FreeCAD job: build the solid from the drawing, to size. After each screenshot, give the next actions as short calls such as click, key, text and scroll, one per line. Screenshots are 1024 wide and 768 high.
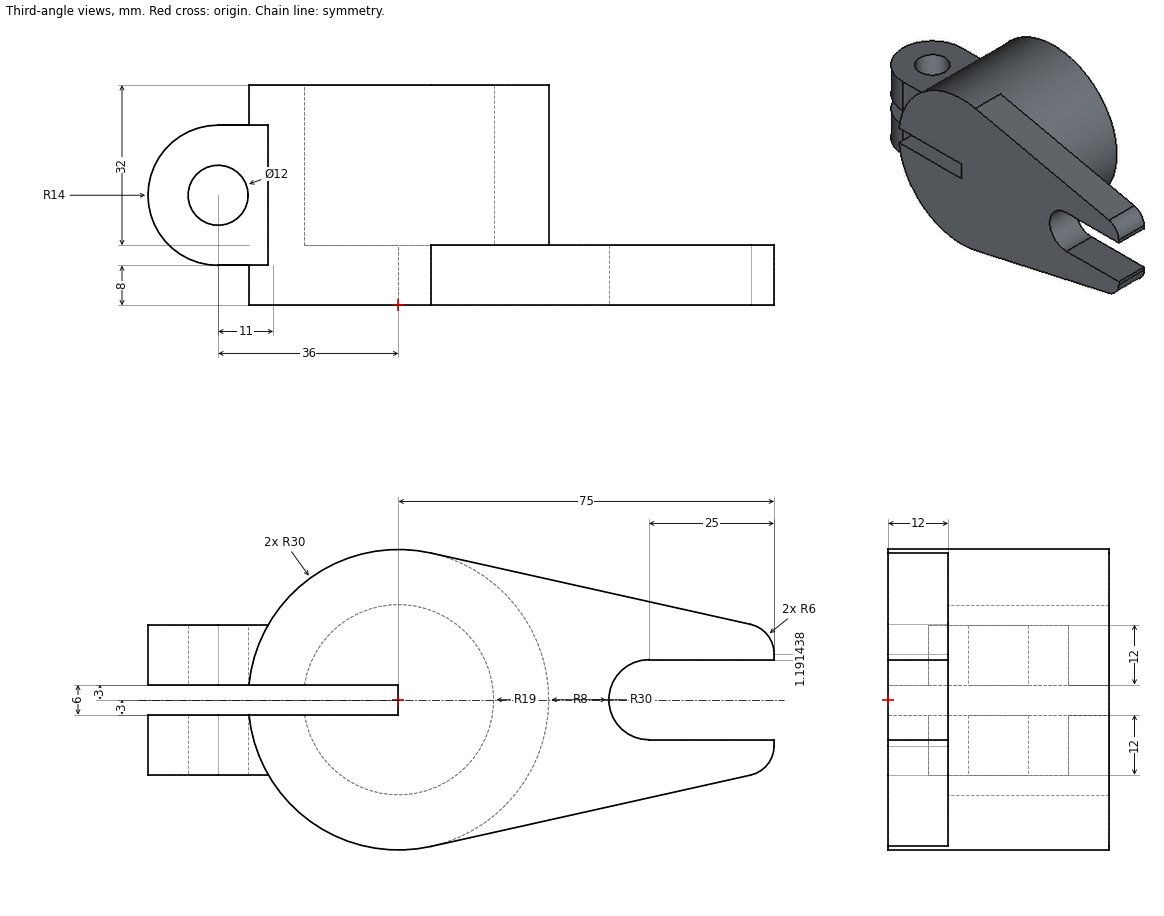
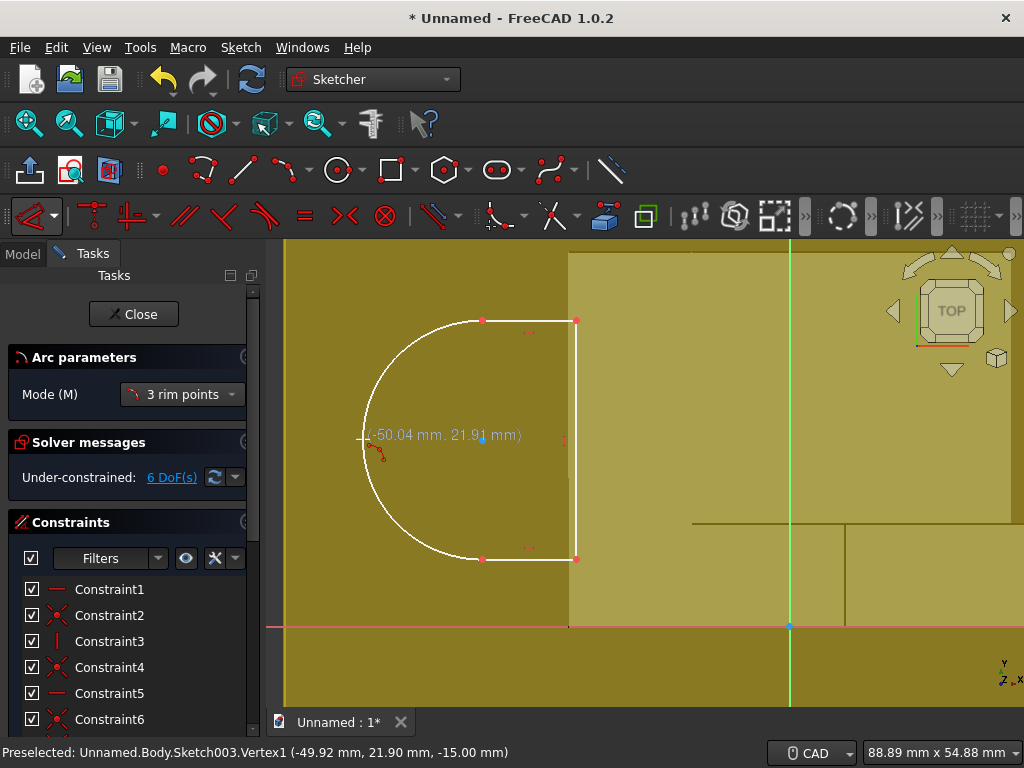
key(g)
key(c)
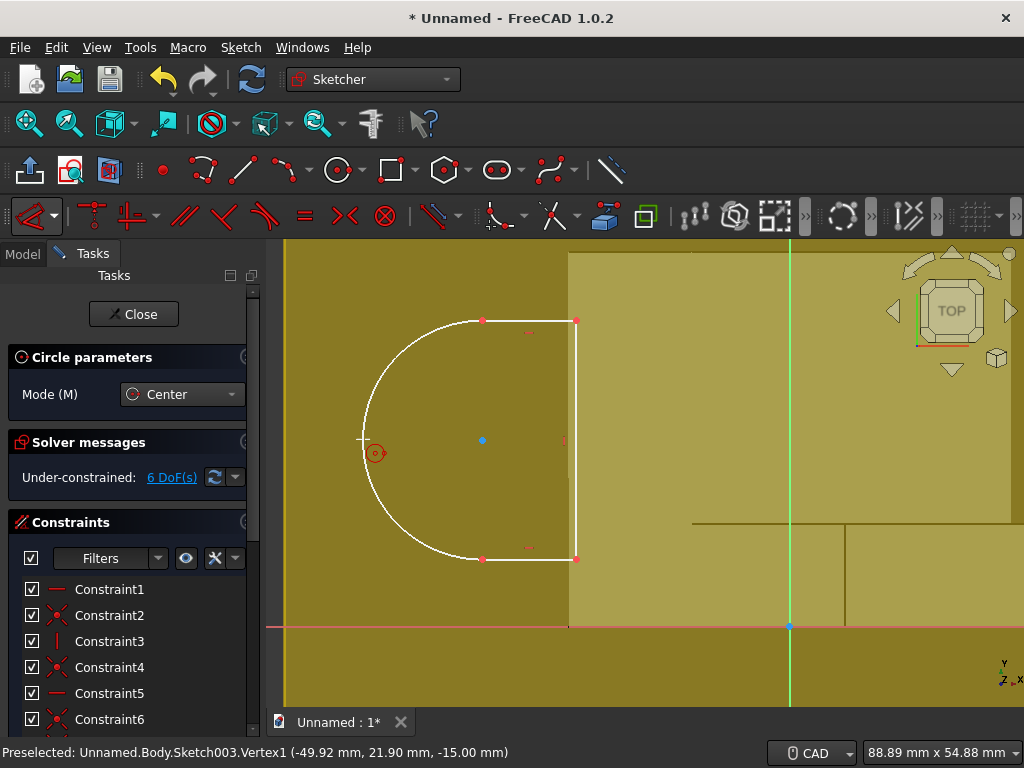
click(483, 439)
click(519, 403)
key(Escape)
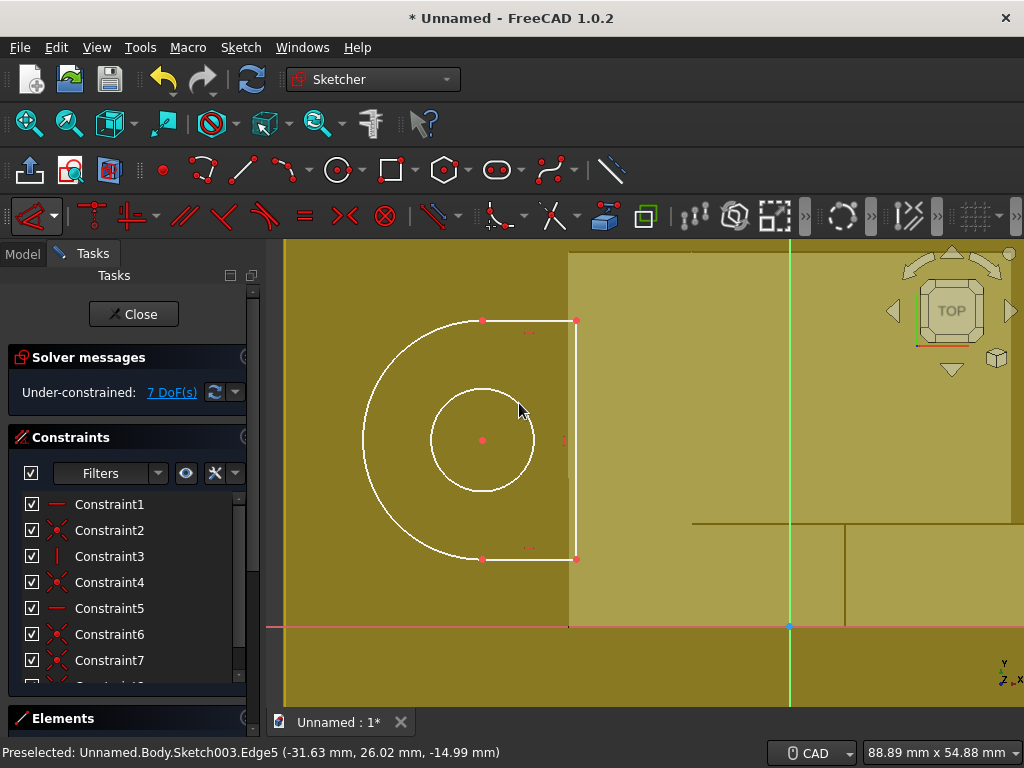
click(511, 560)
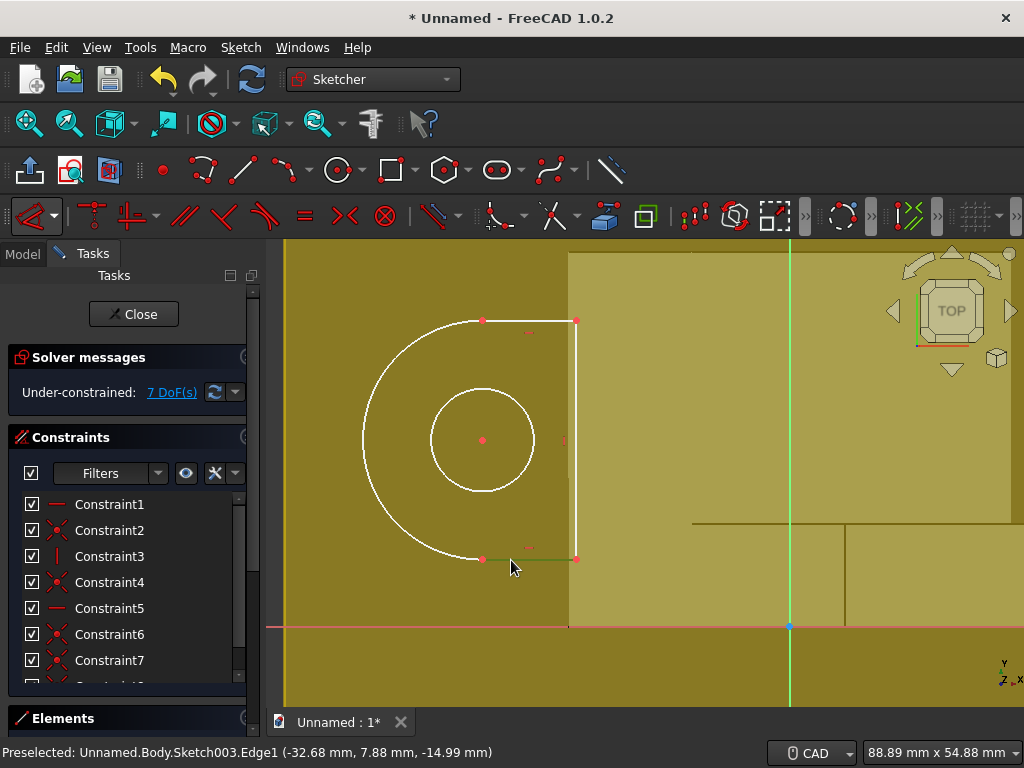
click(386, 370)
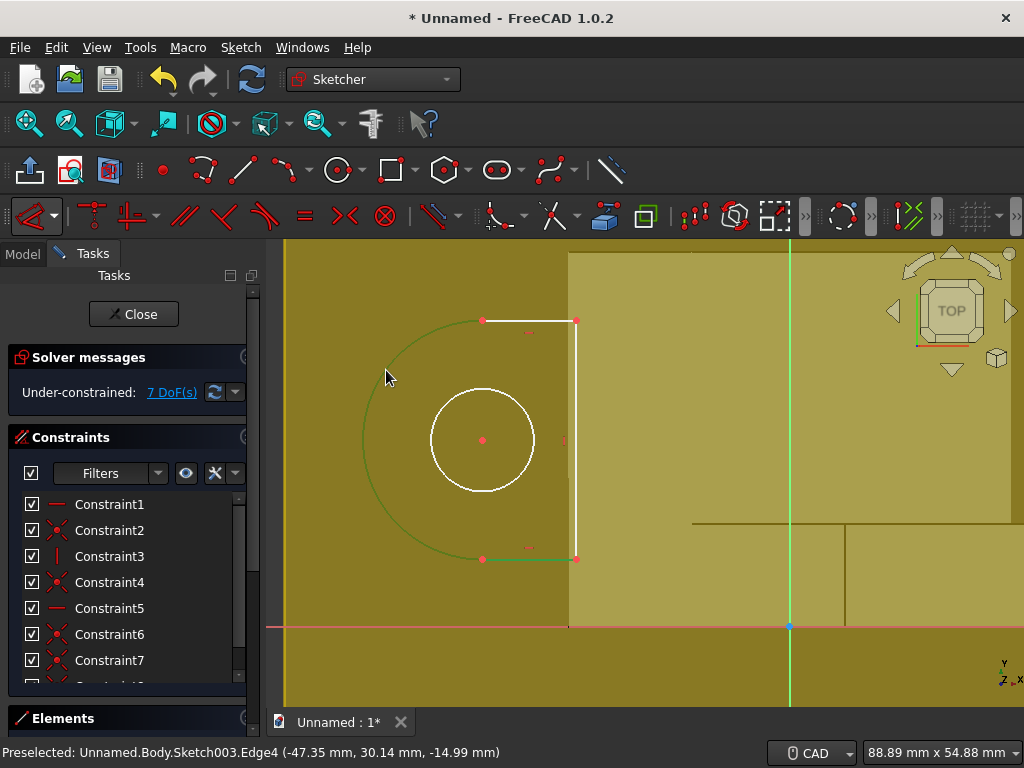
click(266, 216)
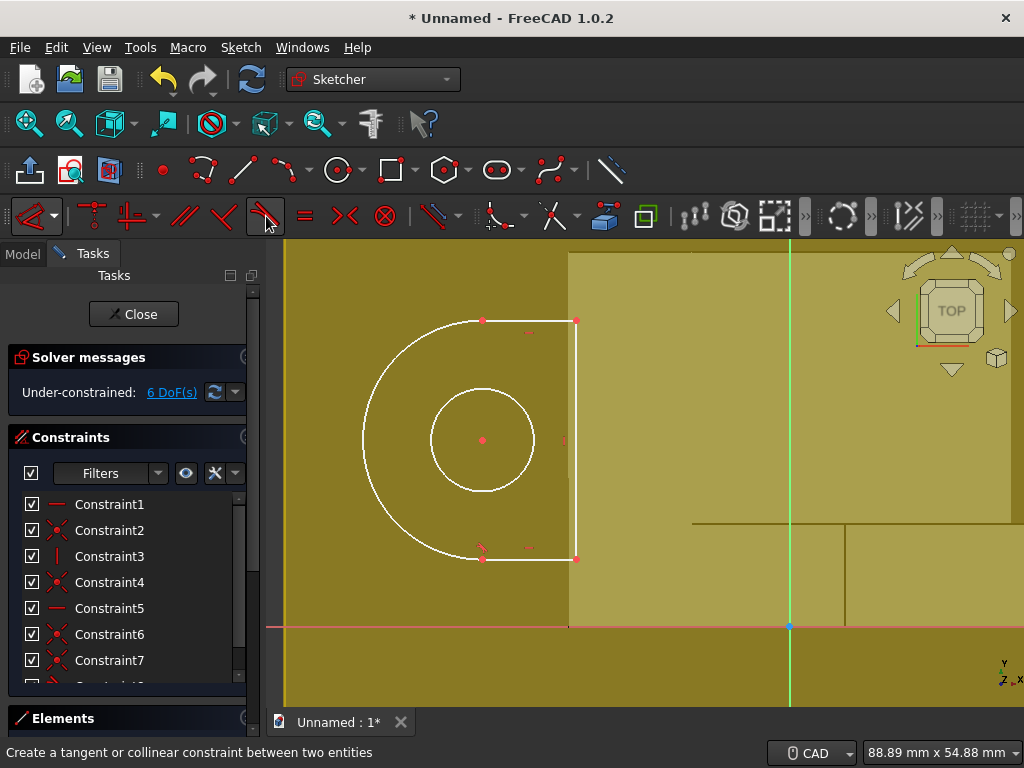
click(548, 321)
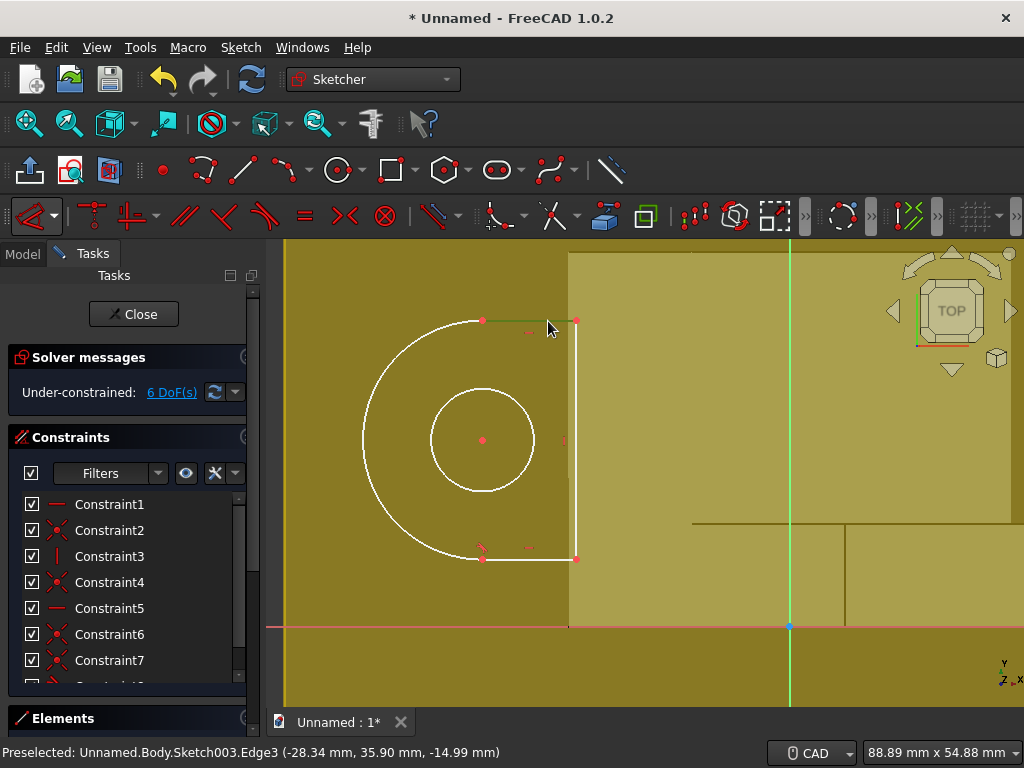
click(386, 370)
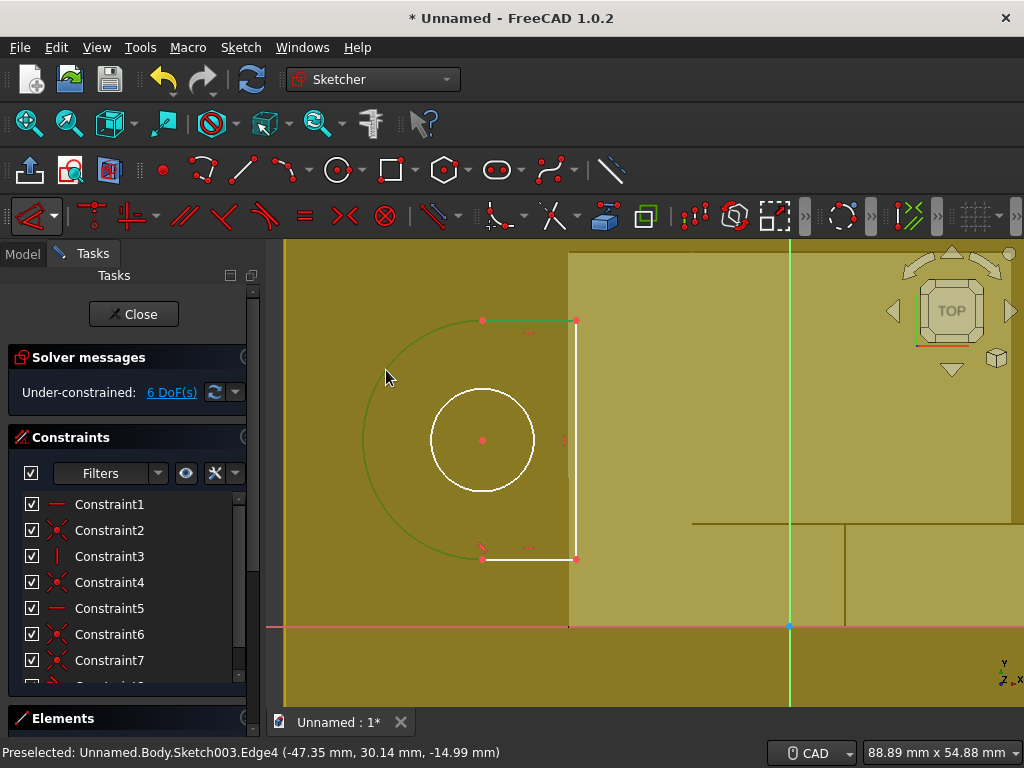
key(t)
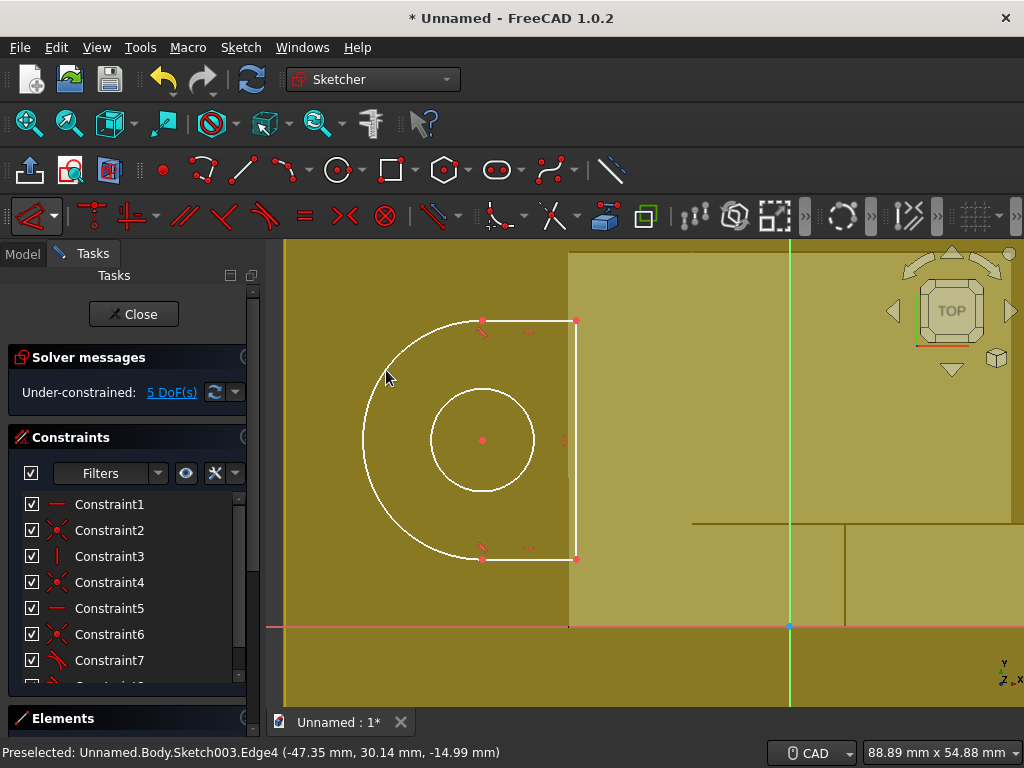
click(386, 370)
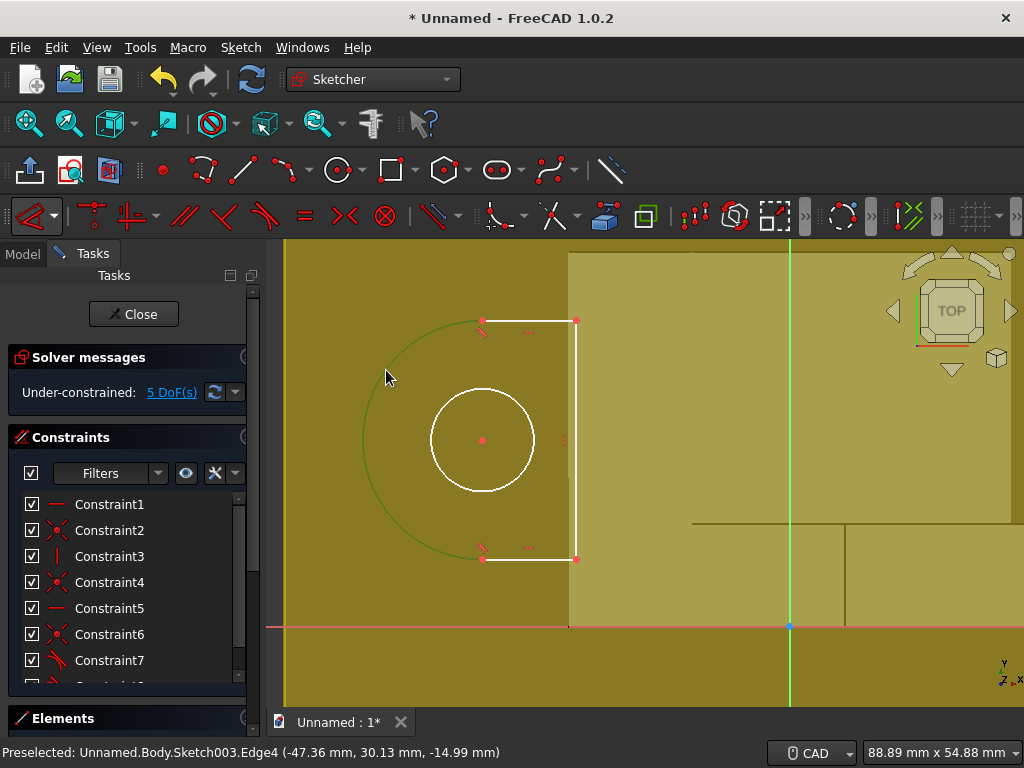
key(k)
key(r)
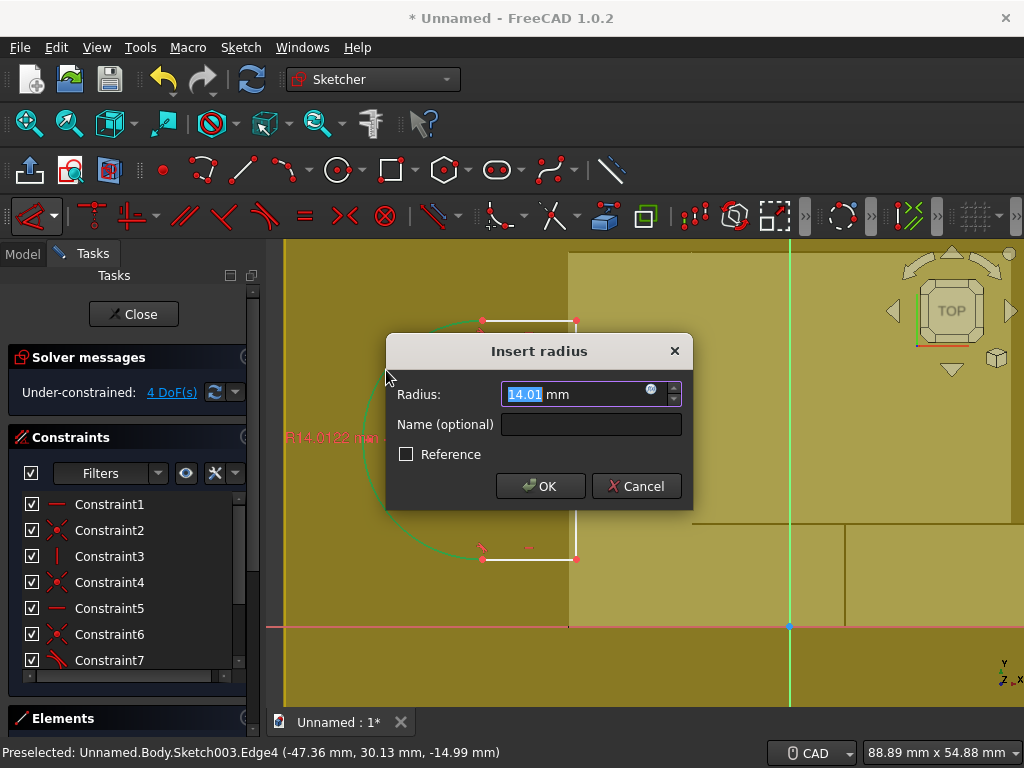
text(14)
key(Return)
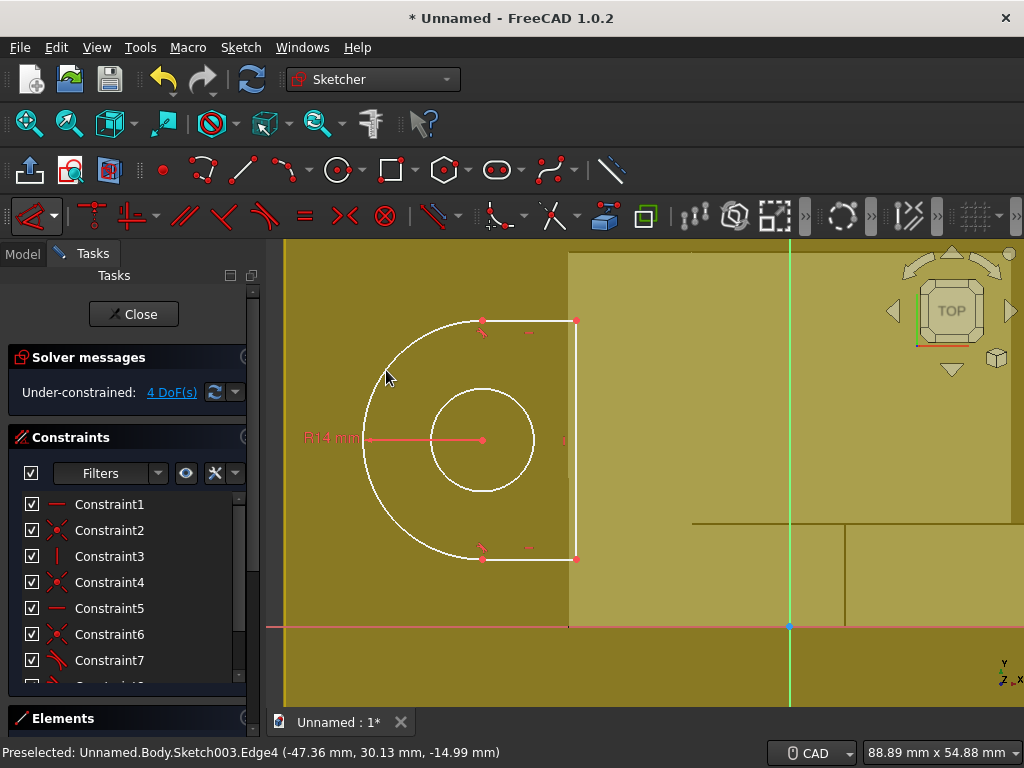
click(519, 404)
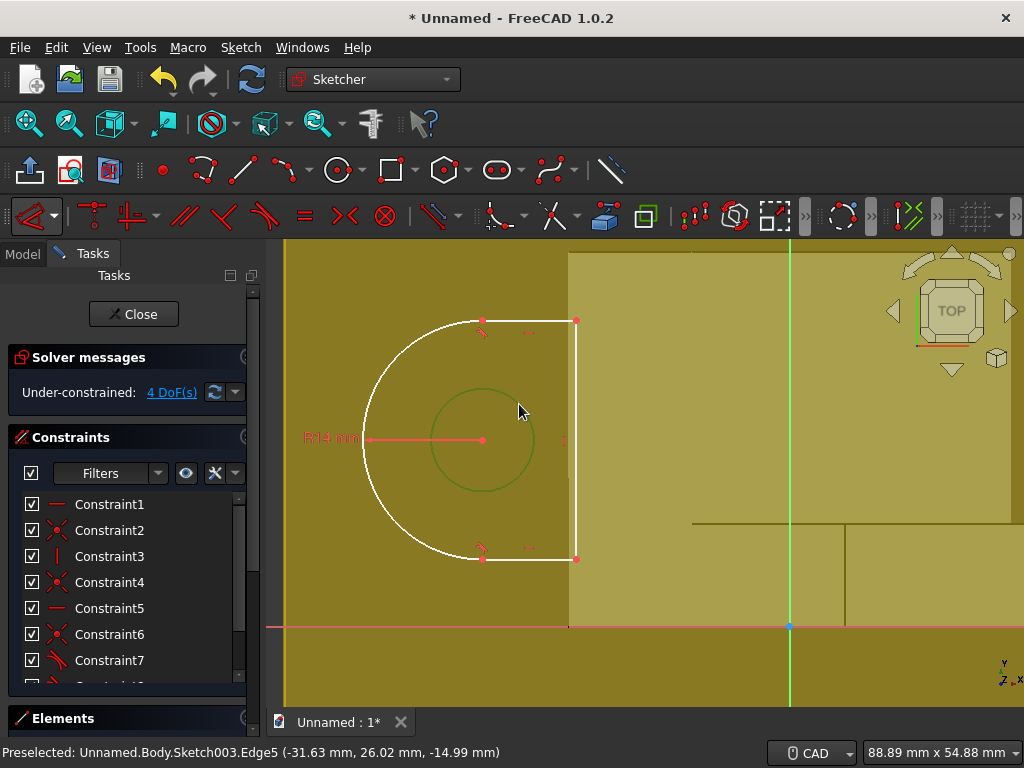
click(56, 216)